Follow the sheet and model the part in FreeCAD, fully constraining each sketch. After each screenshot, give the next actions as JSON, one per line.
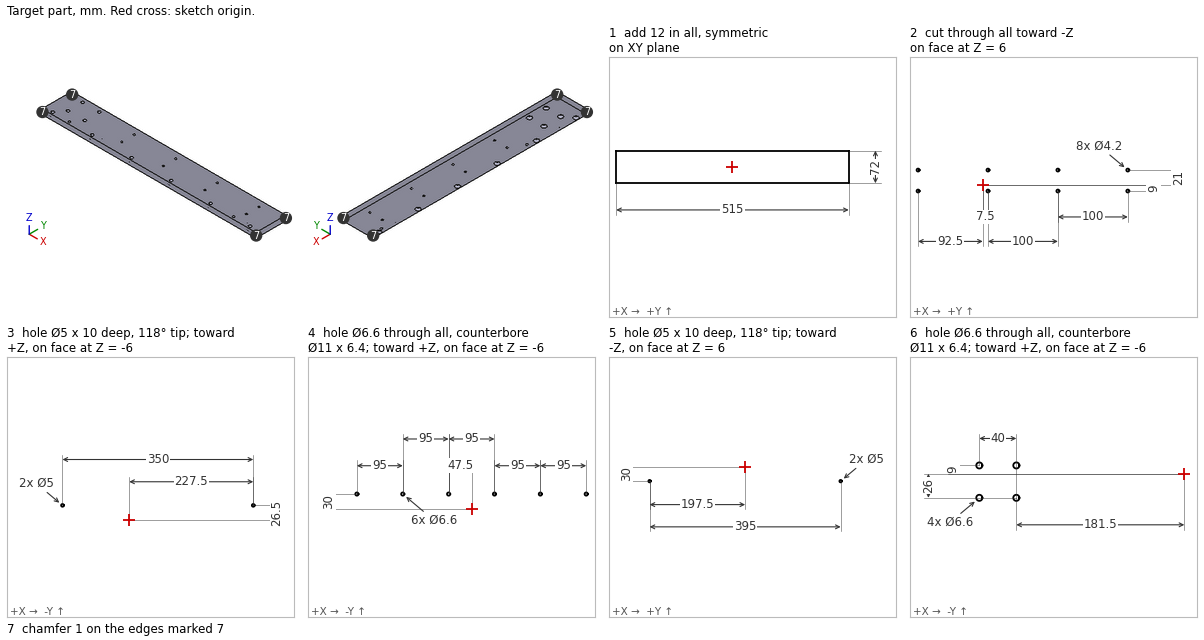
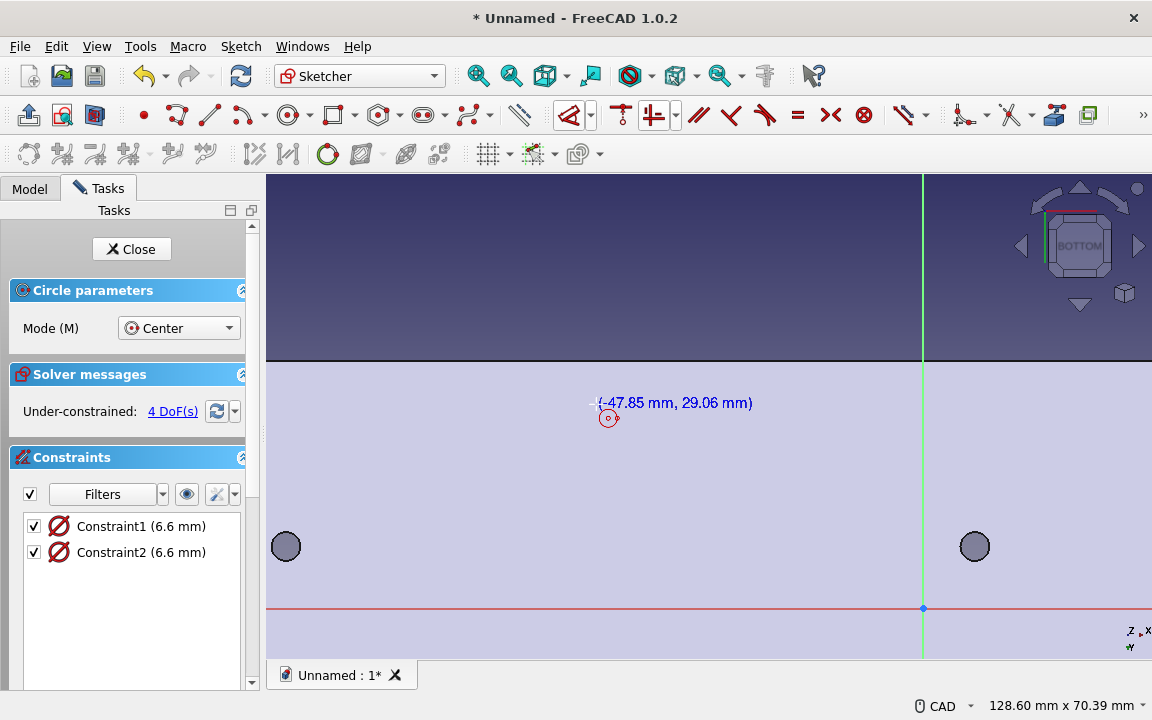
{"action": "scroll", "coordinate": [596, 404], "scroll_direction": "down", "scroll_amount": 10}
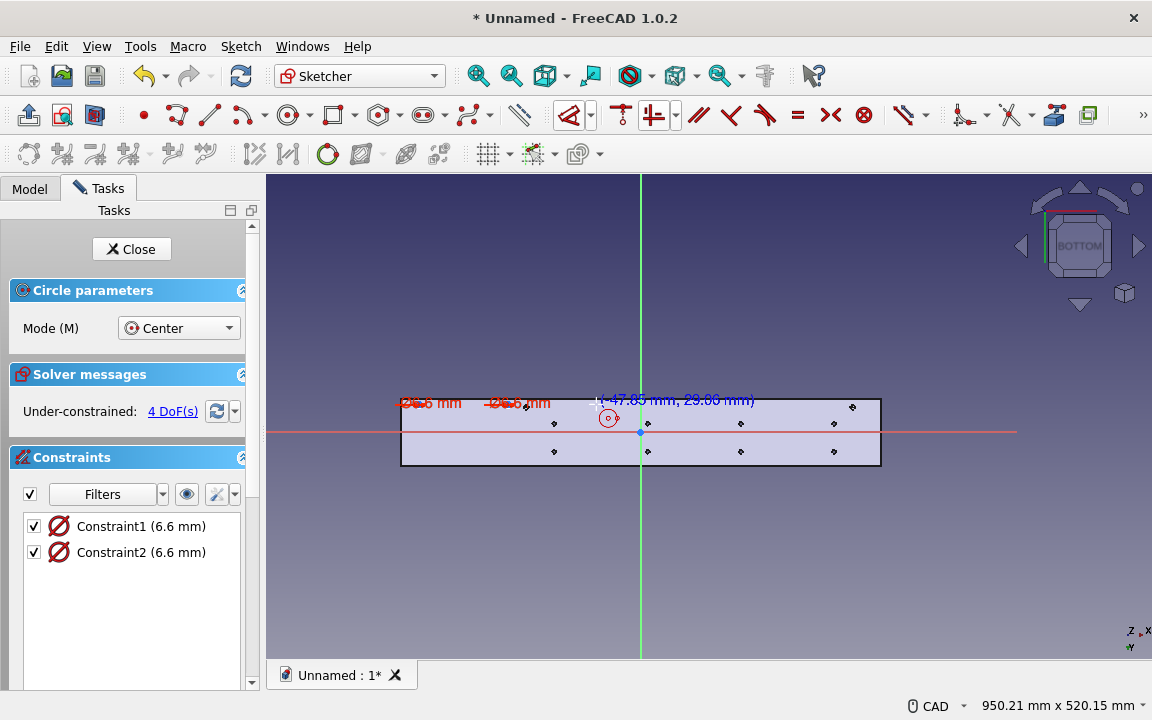
{"action": "left_click", "coordinate": [596, 404]}
{"action": "mouse_move", "coordinate": [598, 402]}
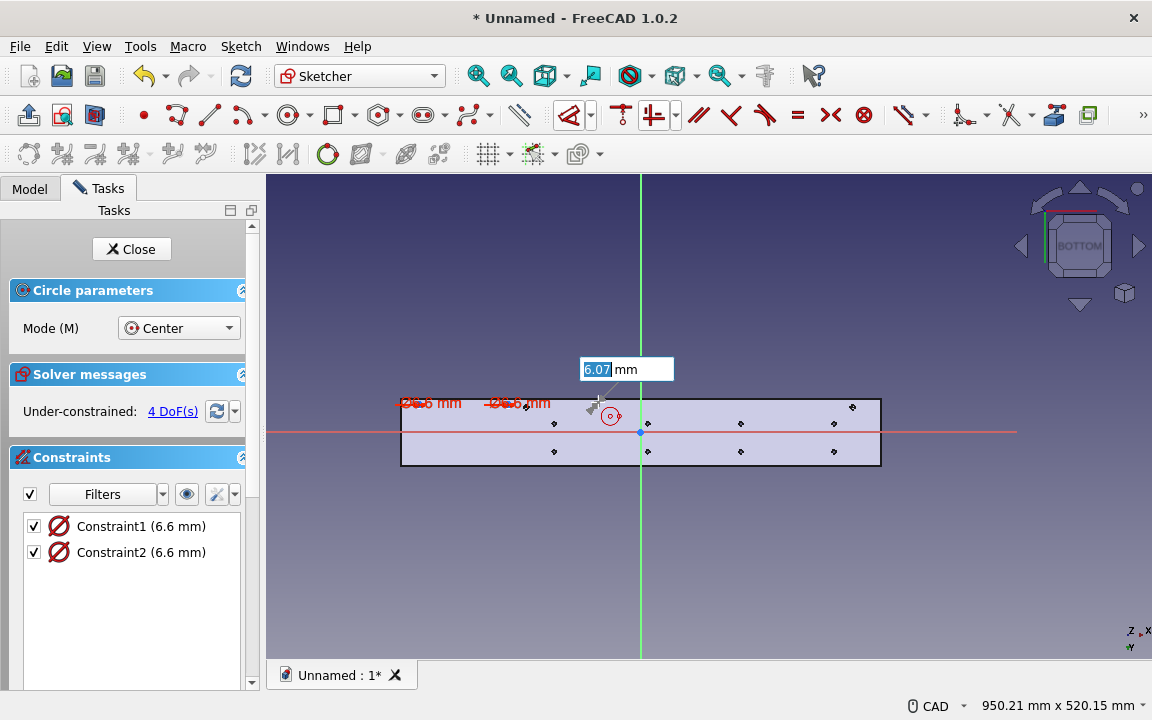
{"action": "type", "text": "6.6"}
{"action": "key", "text": "Return"}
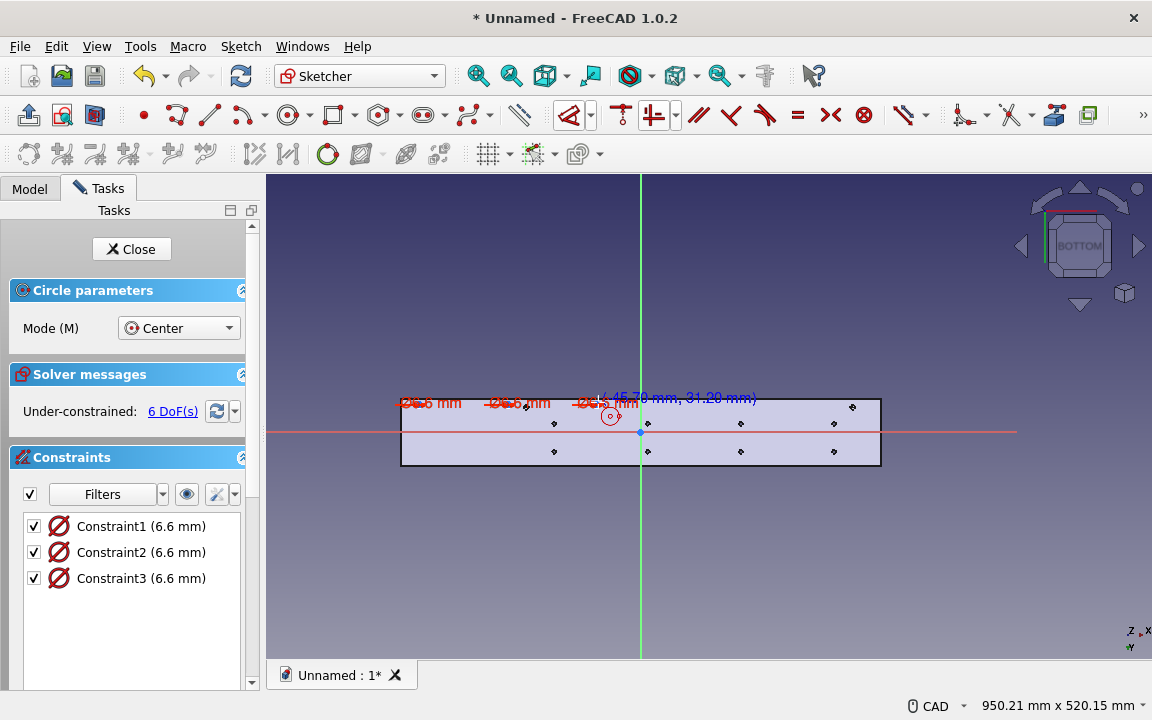
{"action": "scroll", "coordinate": [685, 404], "scroll_direction": "up", "scroll_amount": 10}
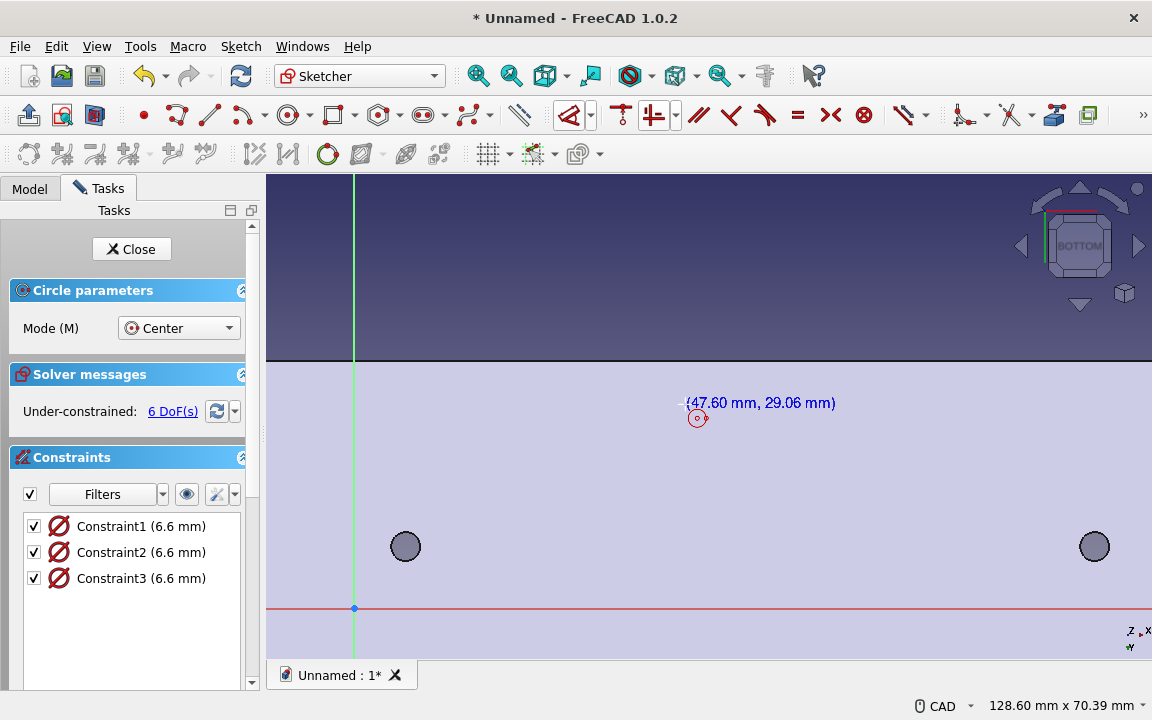
{"action": "scroll", "coordinate": [685, 404], "scroll_direction": "down", "scroll_amount": 10}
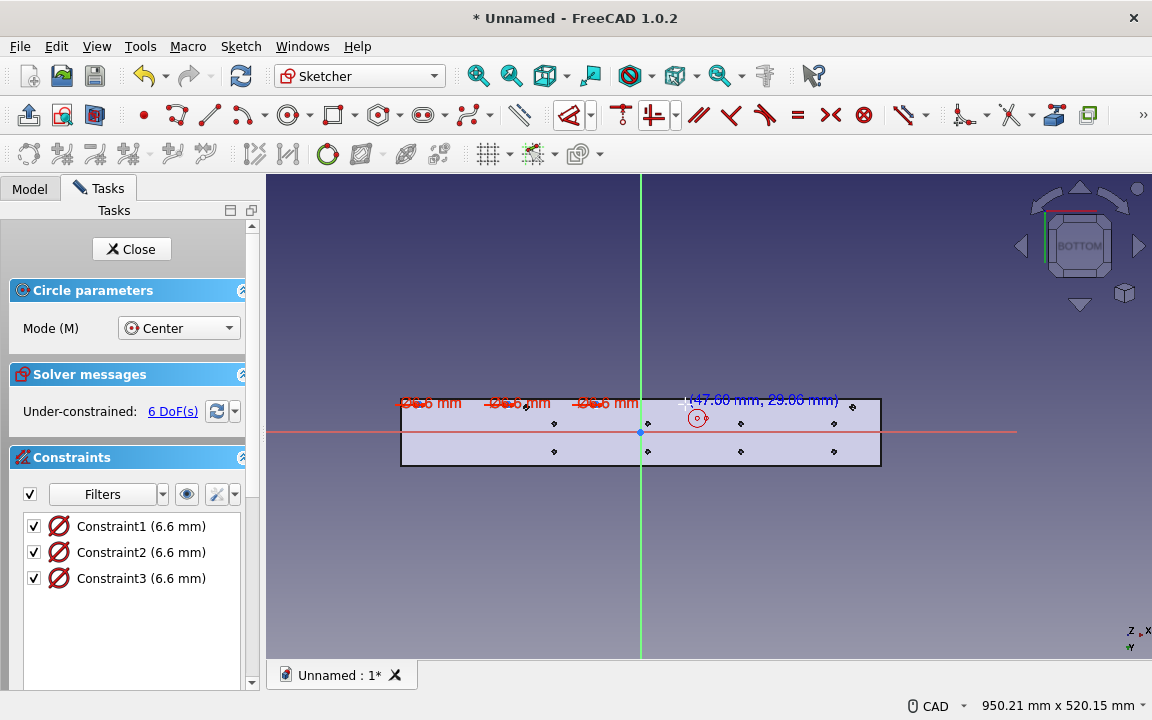
{"action": "left_click", "coordinate": [685, 404]}
{"action": "mouse_move", "coordinate": [687, 402]}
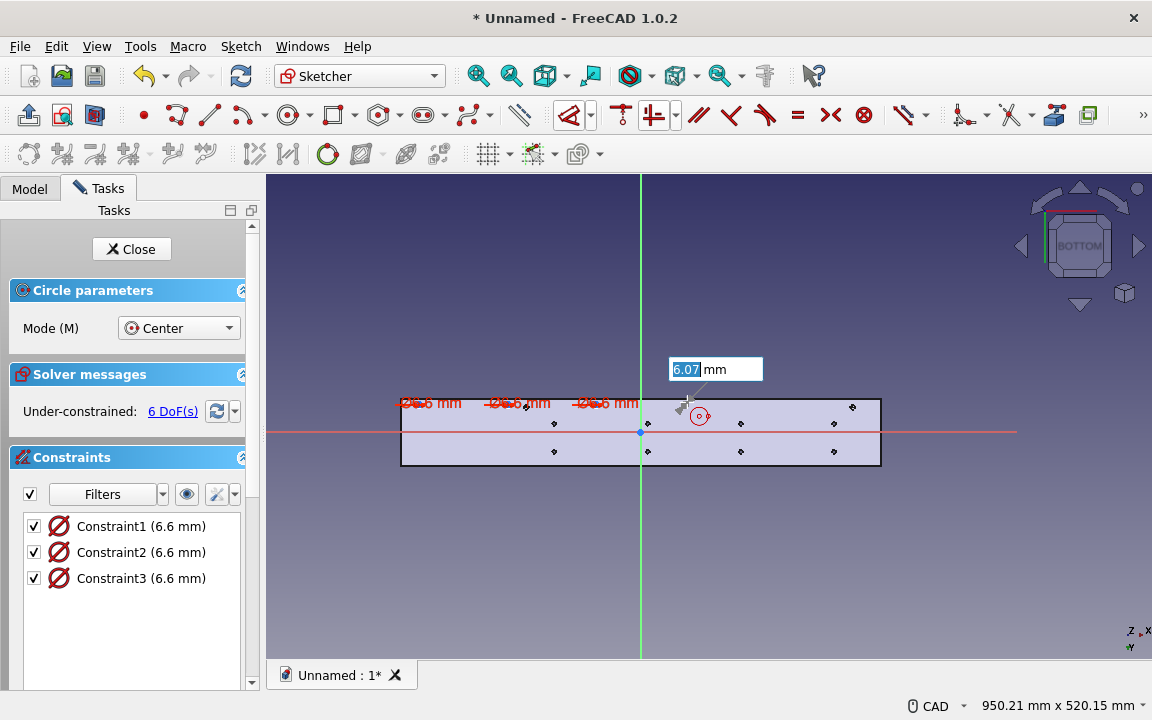
{"action": "type", "text": "6.6"}
{"action": "key", "text": "Return"}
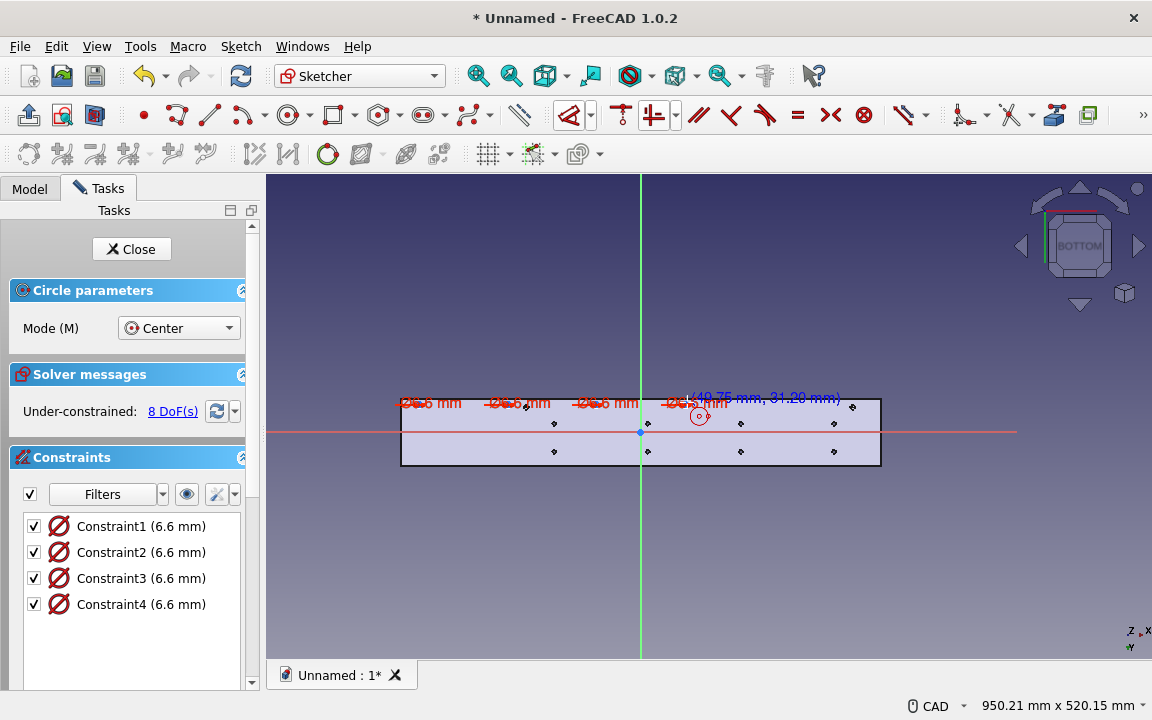
{"action": "scroll", "coordinate": [773, 404], "scroll_direction": "up", "scroll_amount": 10}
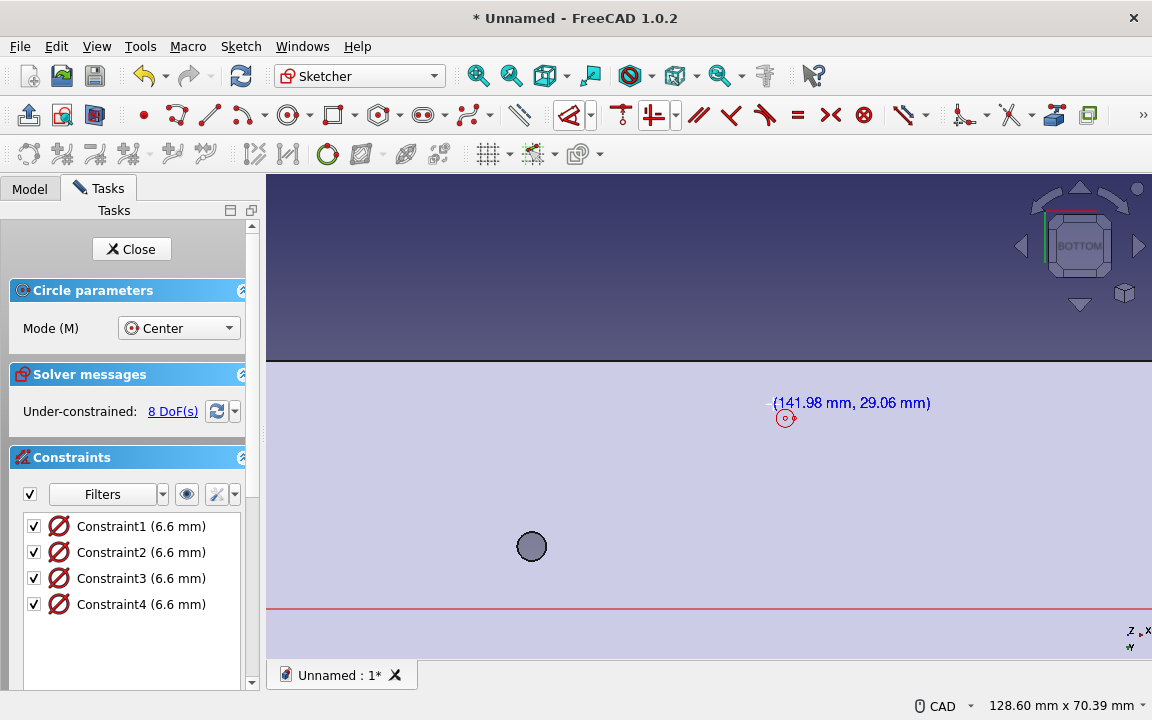
{"action": "scroll", "coordinate": [773, 404], "scroll_direction": "down", "scroll_amount": 10}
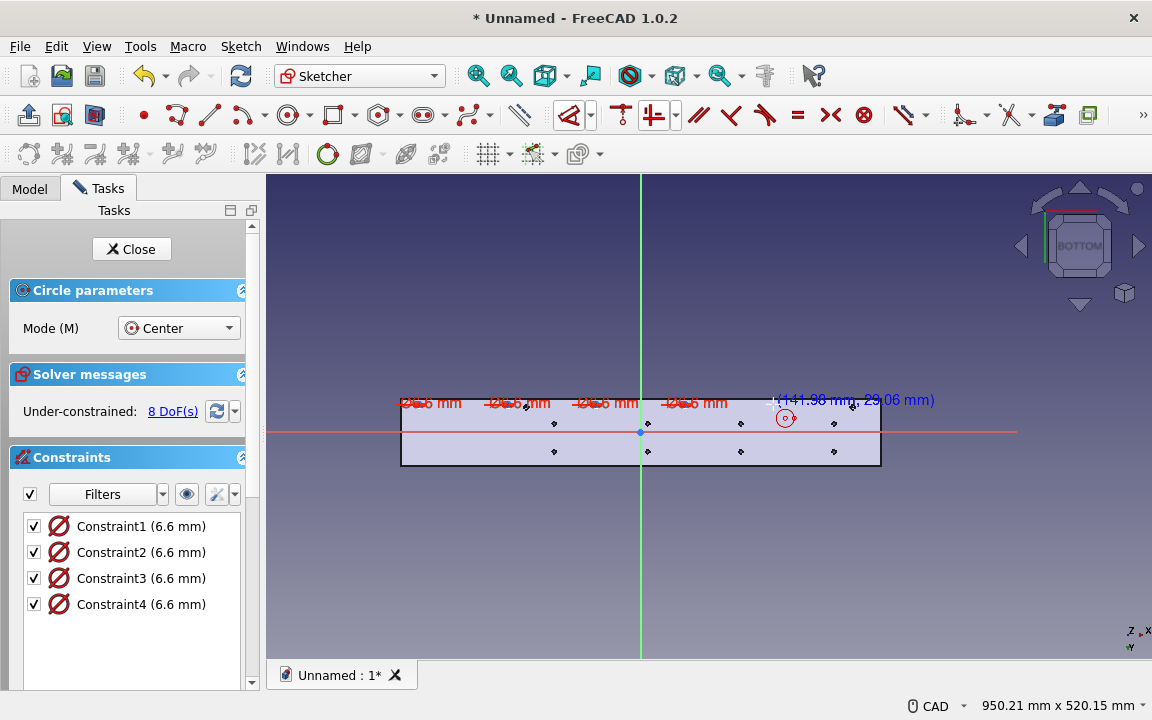
{"action": "left_click", "coordinate": [773, 404]}
{"action": "mouse_move", "coordinate": [776, 402]}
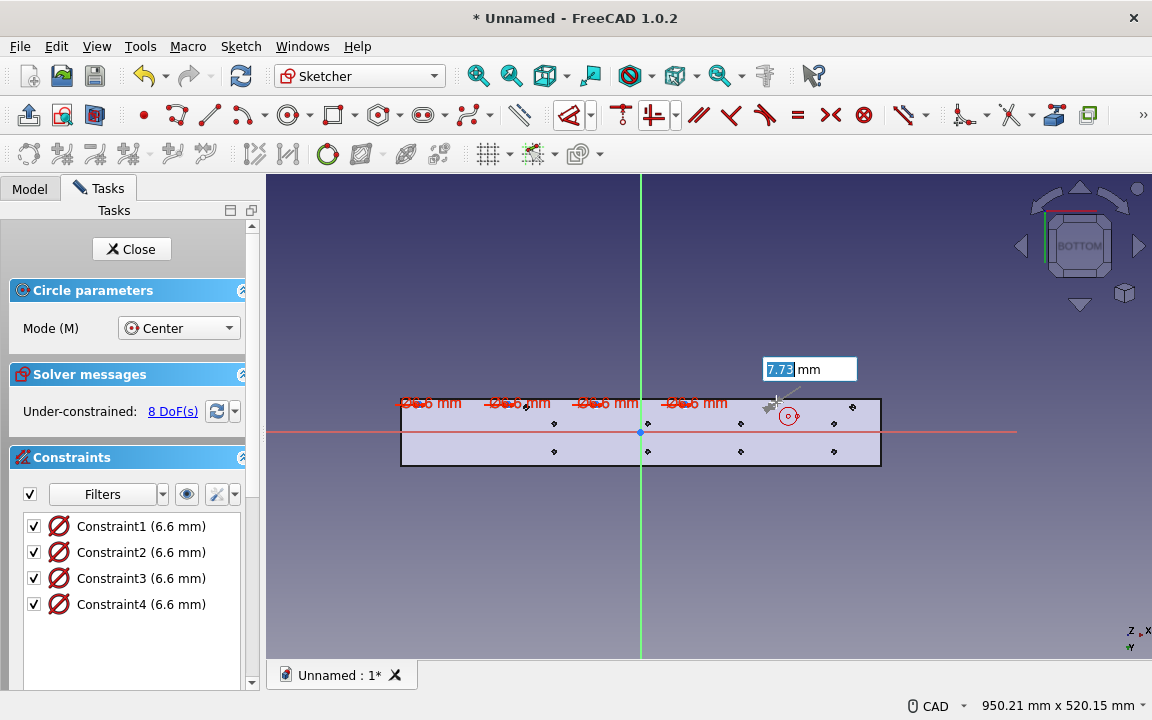
{"action": "type", "text": "6.6"}
{"action": "key", "text": "Return"}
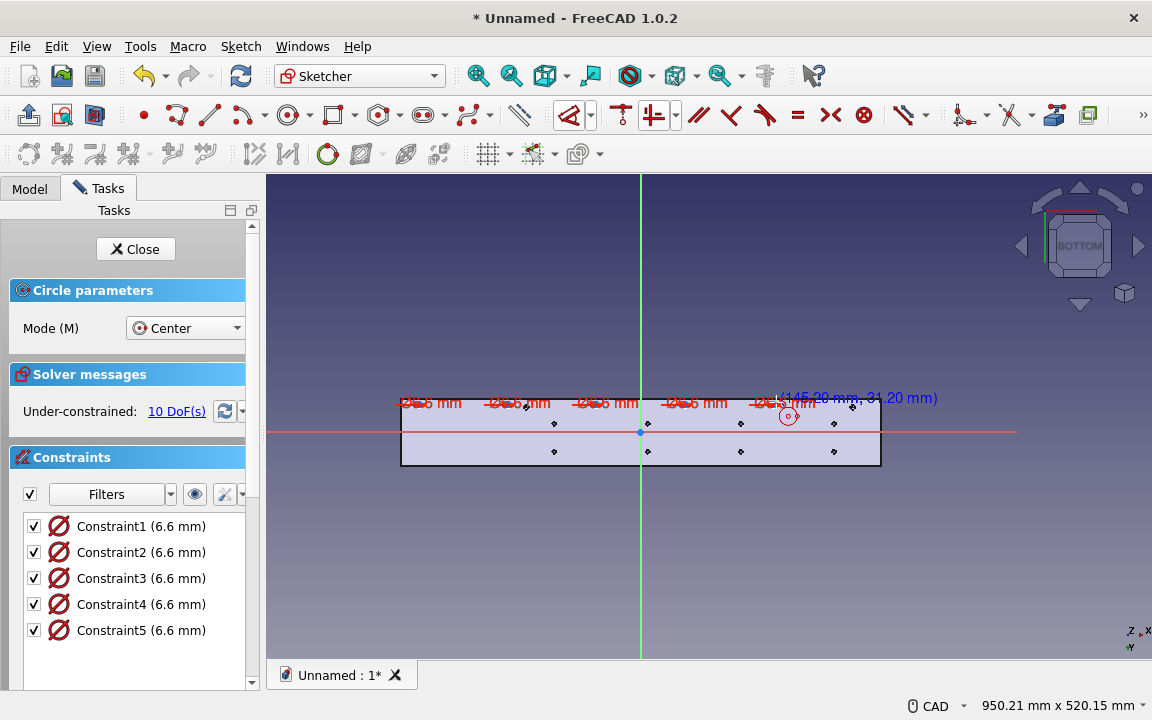
{"action": "scroll", "coordinate": [862, 404], "scroll_direction": "up", "scroll_amount": 10}